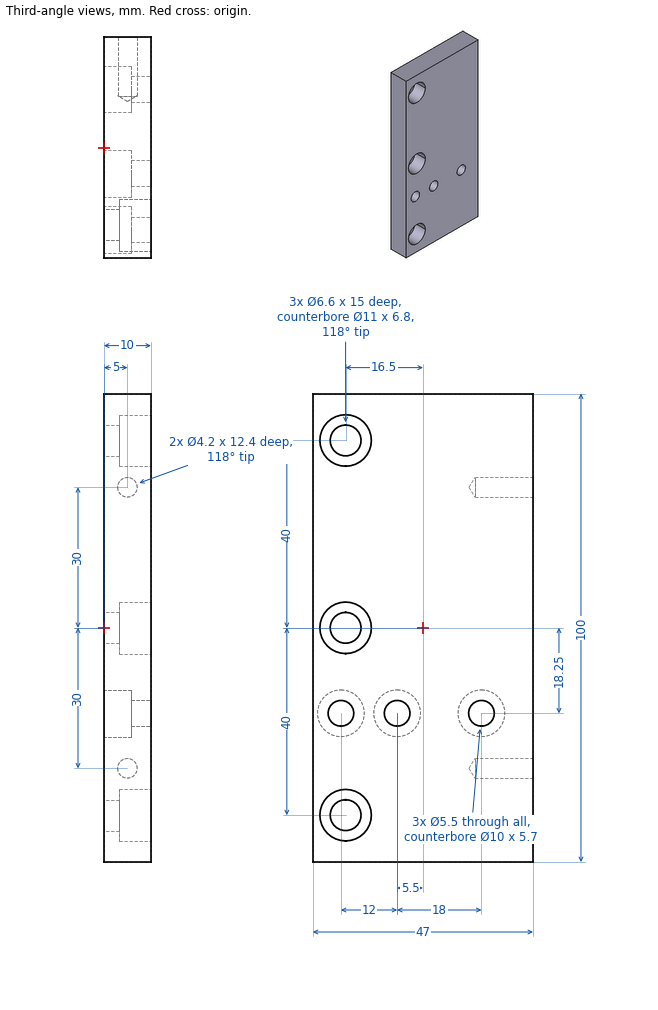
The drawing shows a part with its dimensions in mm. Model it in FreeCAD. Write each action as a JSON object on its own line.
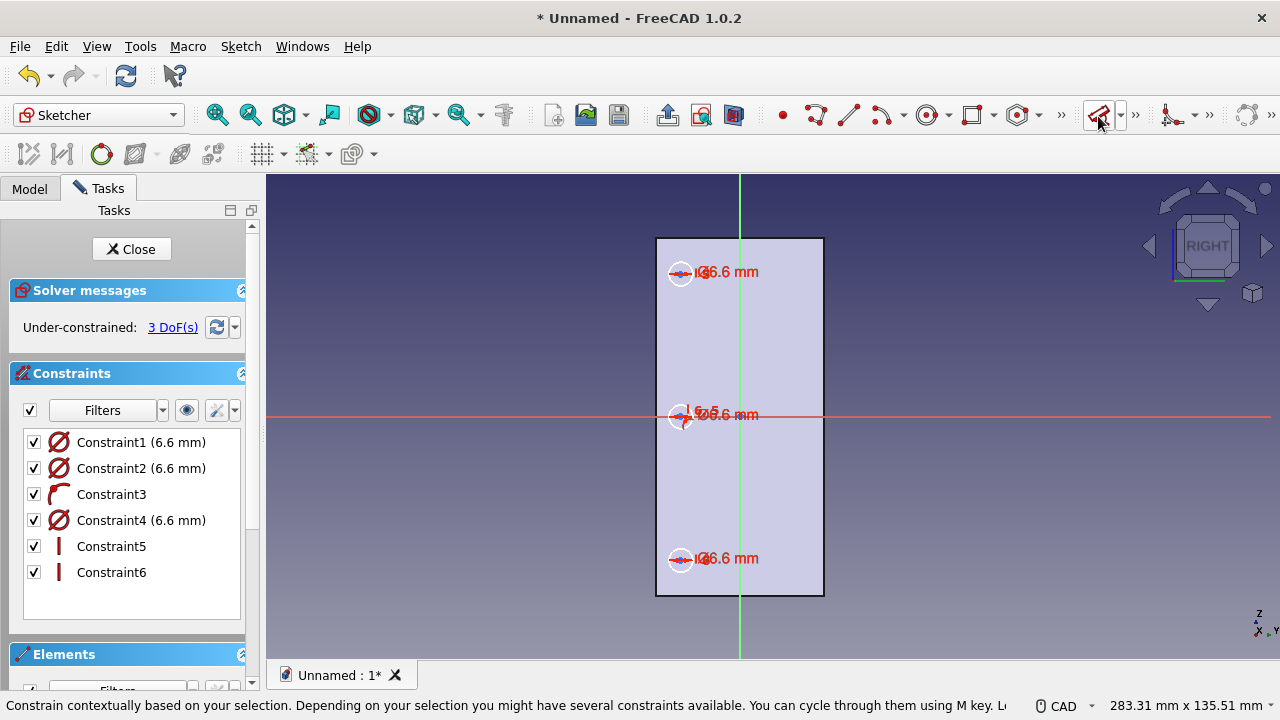
{"action": "left_click", "coordinate": [681, 274]}
{"action": "left_click", "coordinate": [774, 345]}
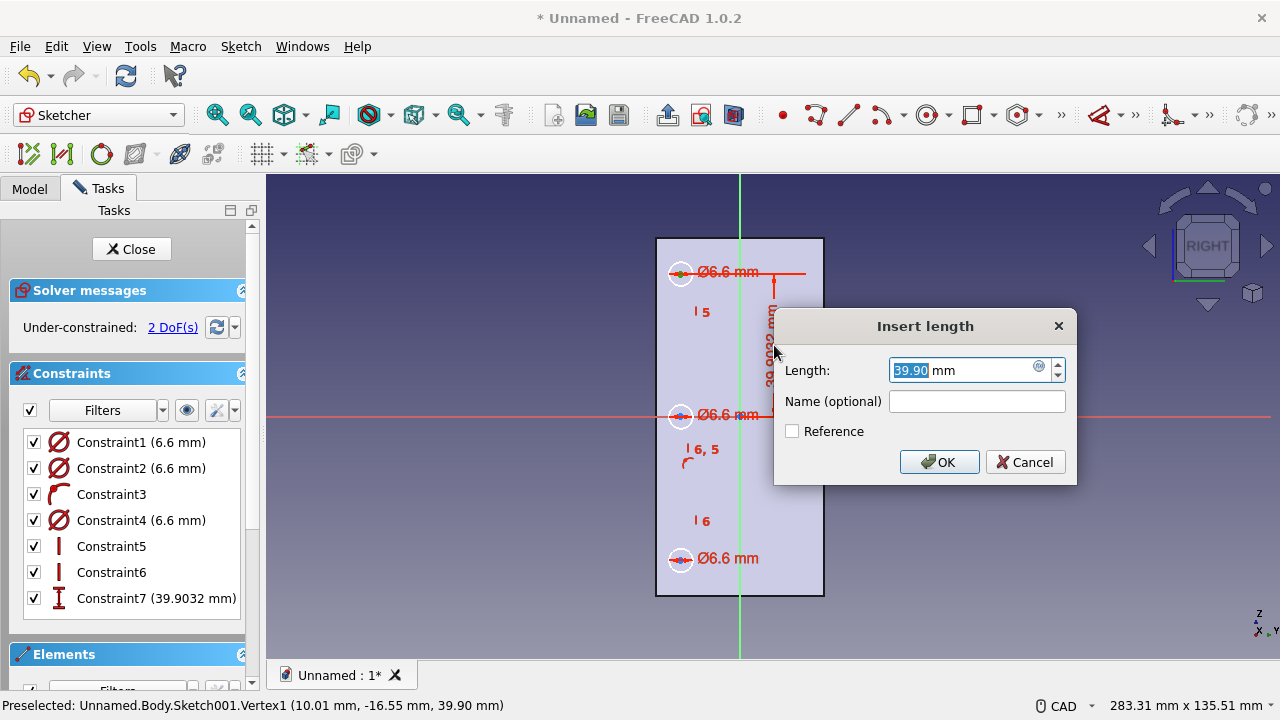
{"action": "type", "text": "40"}
{"action": "key", "text": "Return"}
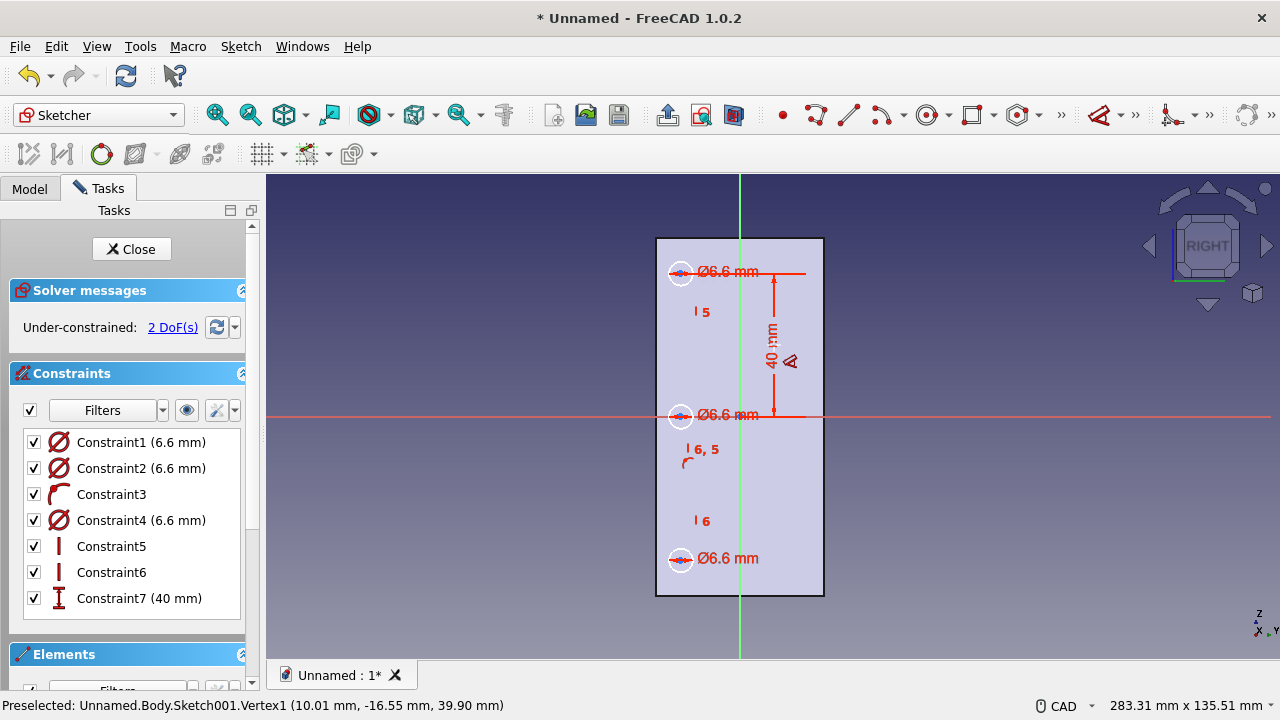
{"action": "left_click", "coordinate": [681, 560]}
{"action": "left_click", "coordinate": [774, 489]}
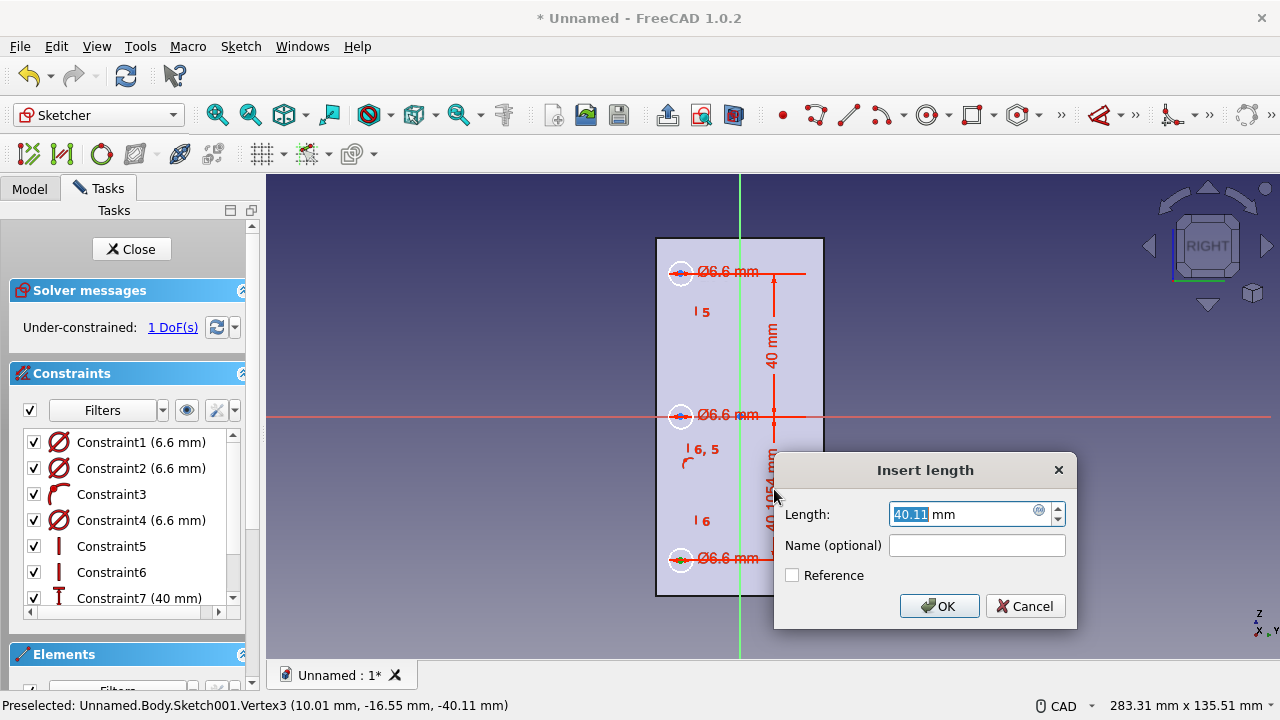
{"action": "type", "text": "40"}
{"action": "key", "text": "Return"}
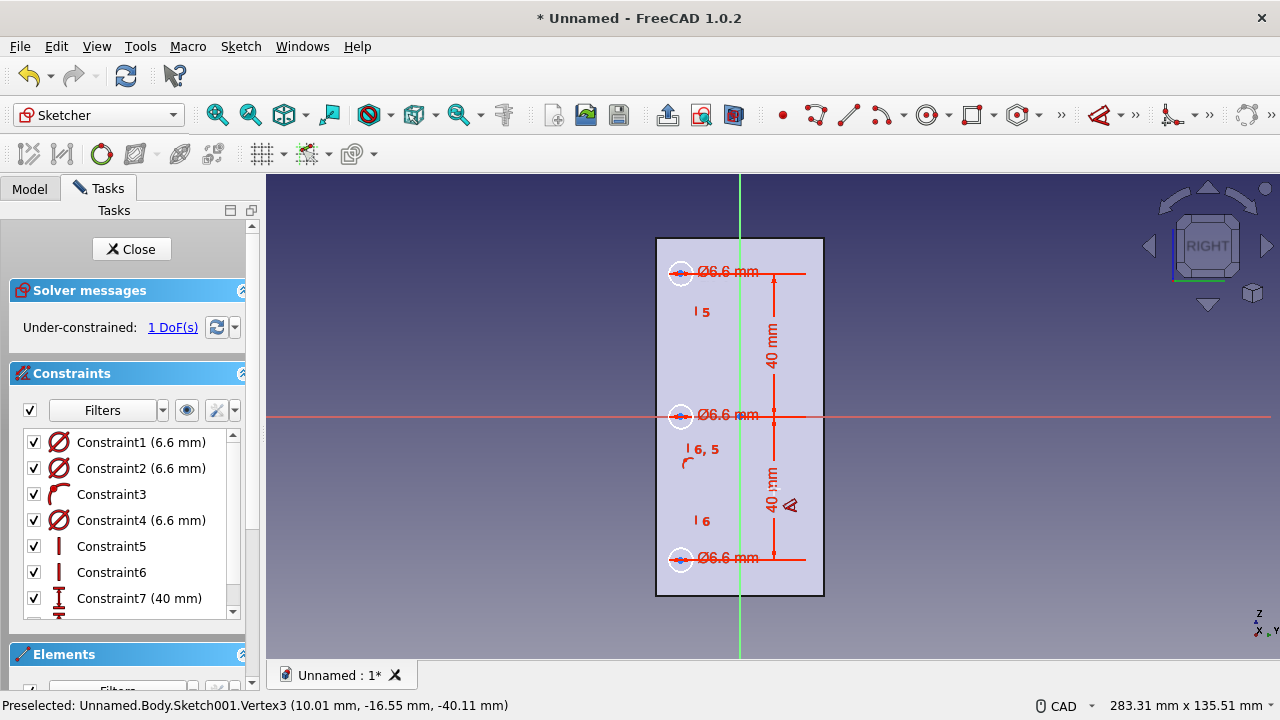
{"action": "left_click", "coordinate": [681, 274]}
{"action": "left_click", "coordinate": [711, 240]}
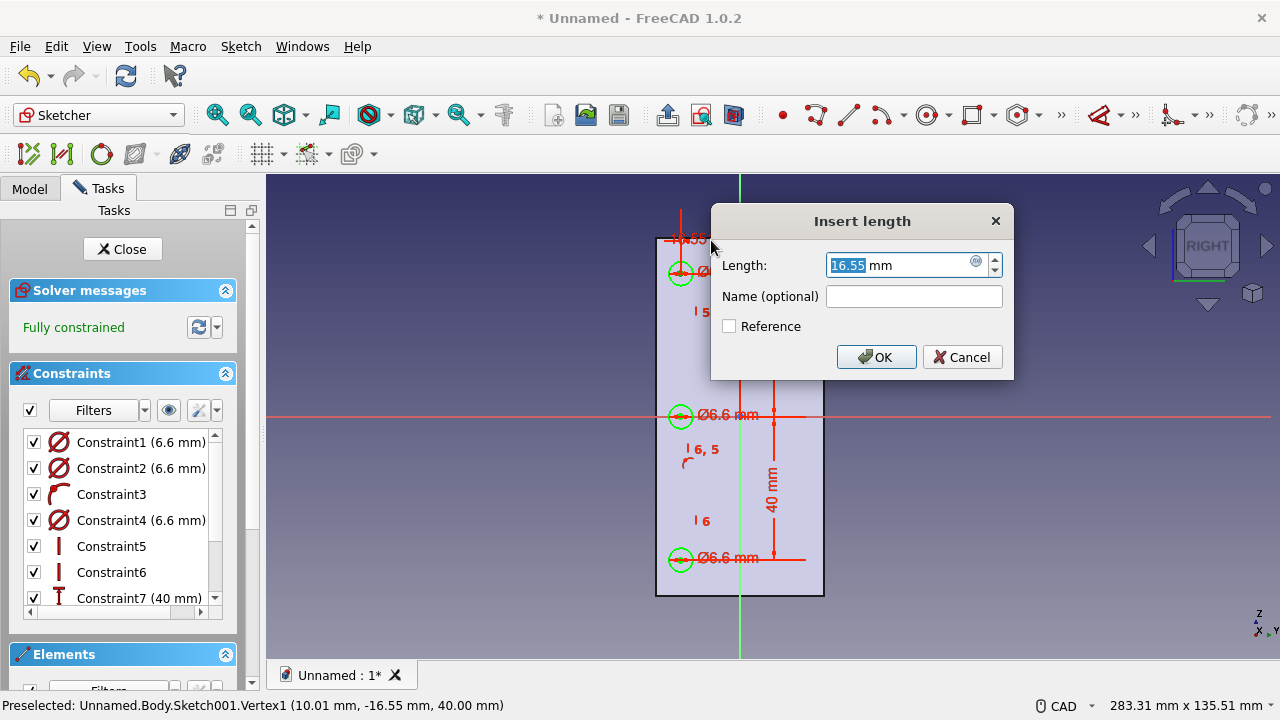
{"action": "type", "text": "16.5"}
{"action": "key", "text": "Return"}
{"action": "key", "text": "Escape"}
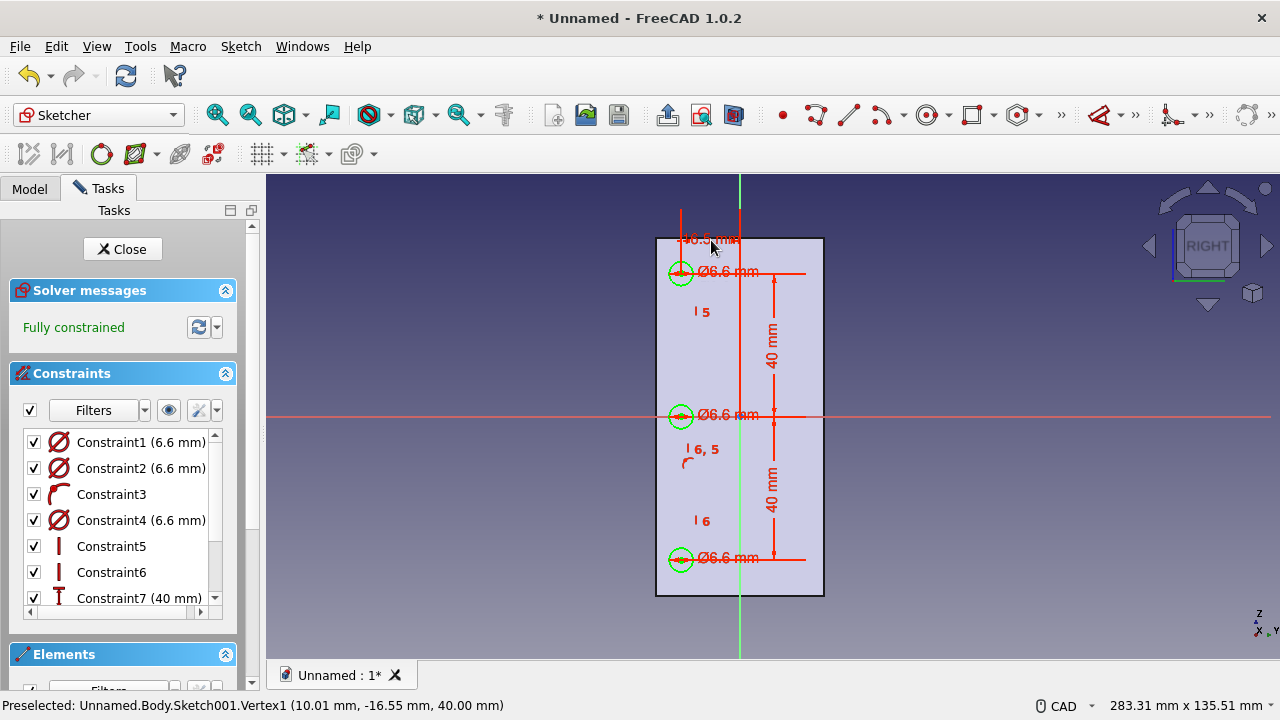
{"action": "left_click", "coordinate": [123, 249]}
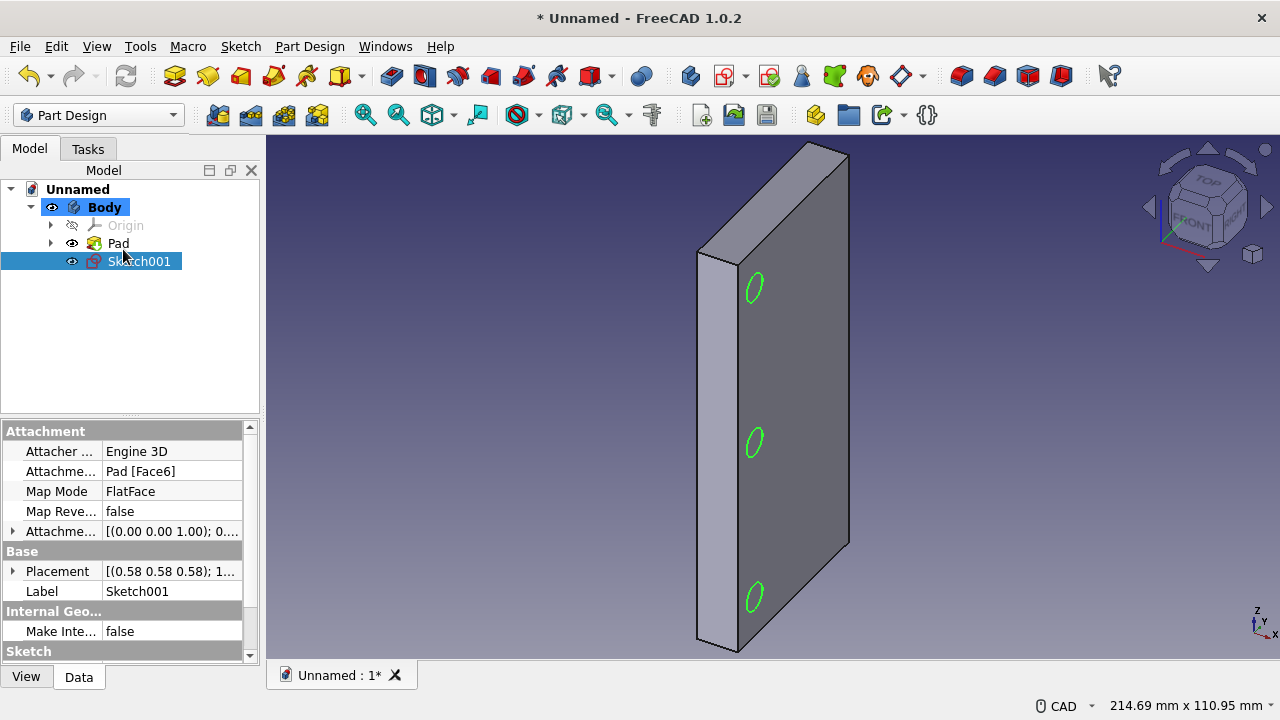
{"action": "left_click", "coordinate": [425, 76]}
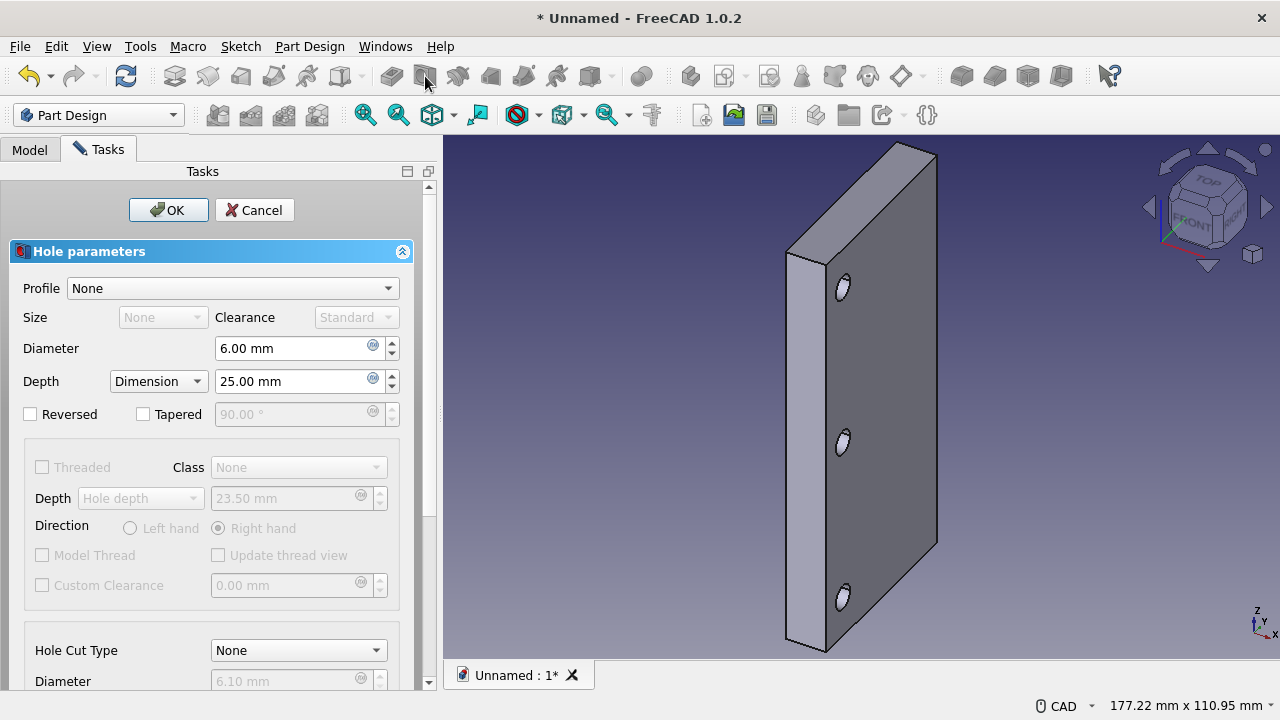
{"action": "triple_click", "coordinate": [300, 348]}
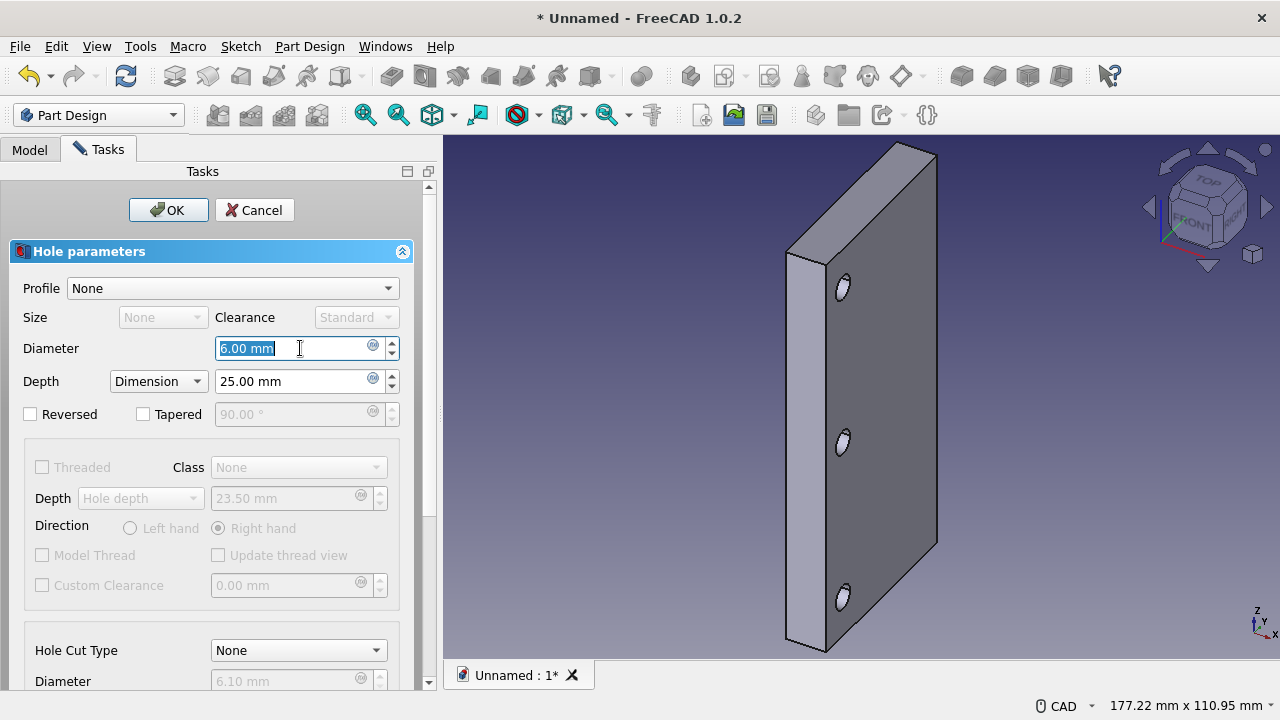
{"action": "type", "text": "6.6"}
{"action": "key", "text": "Tab"}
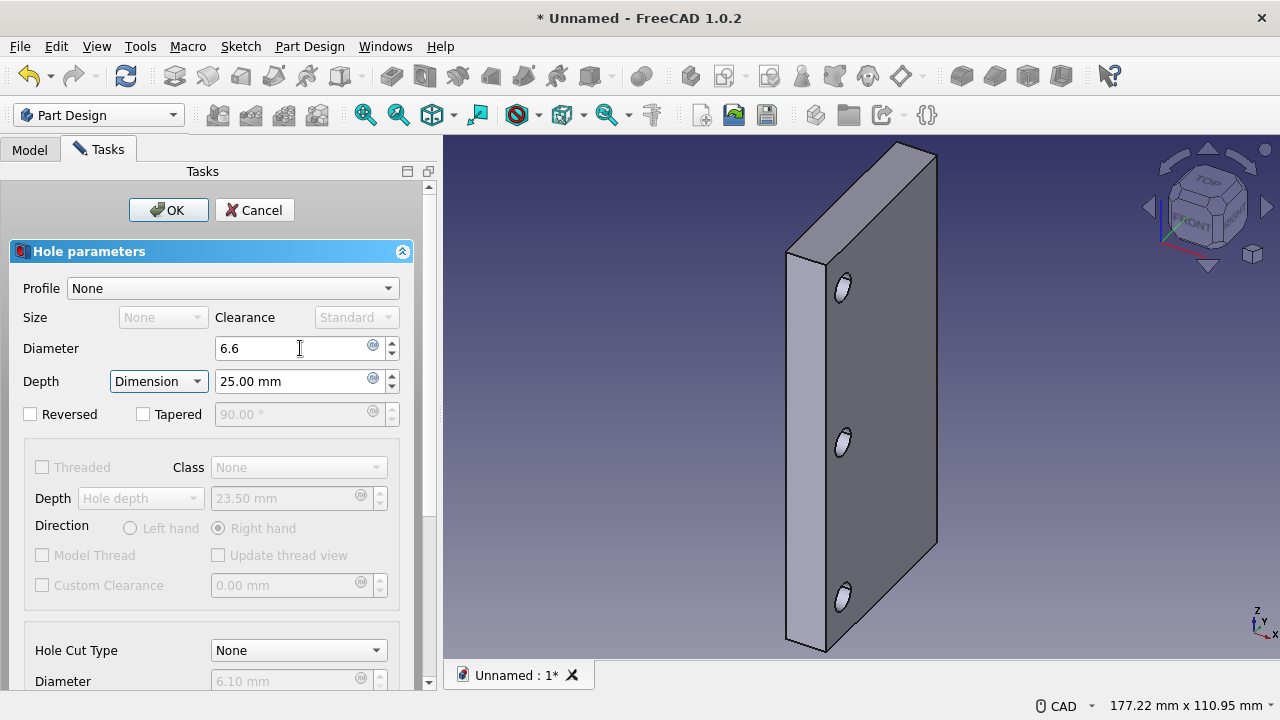
{"action": "triple_click", "coordinate": [300, 382]}